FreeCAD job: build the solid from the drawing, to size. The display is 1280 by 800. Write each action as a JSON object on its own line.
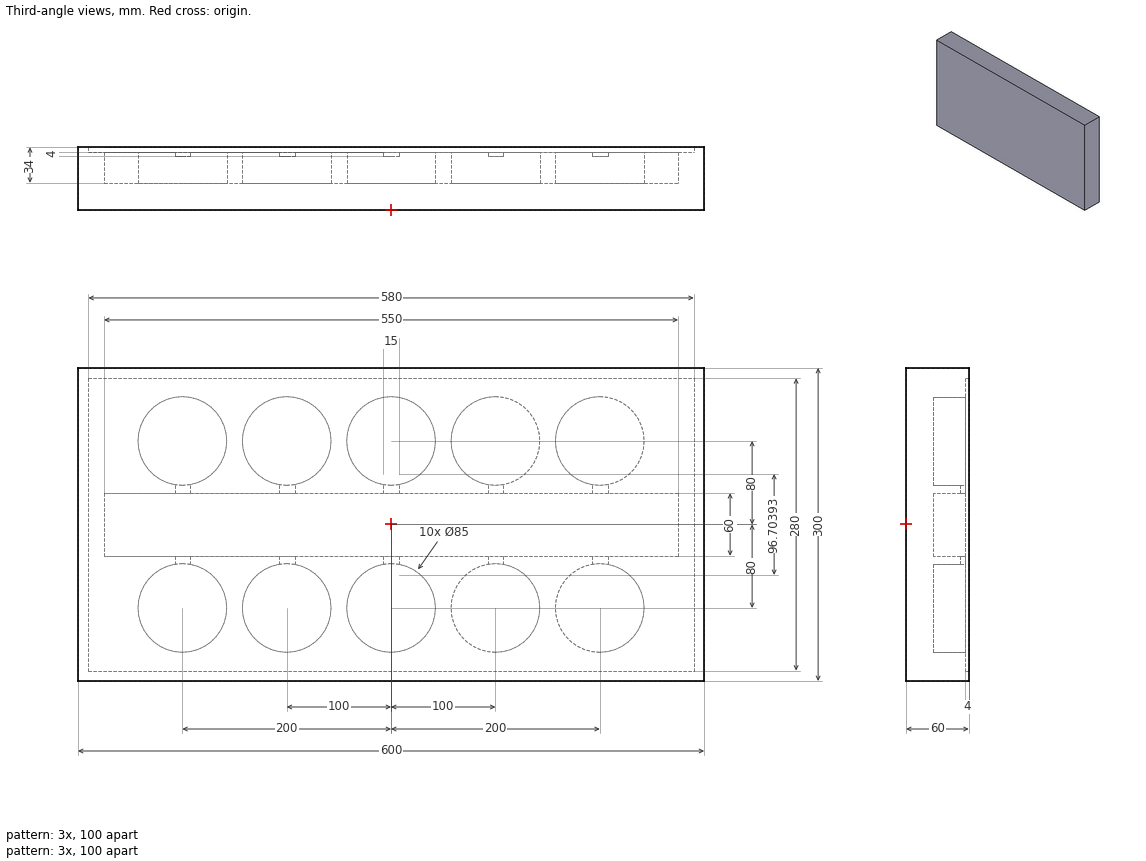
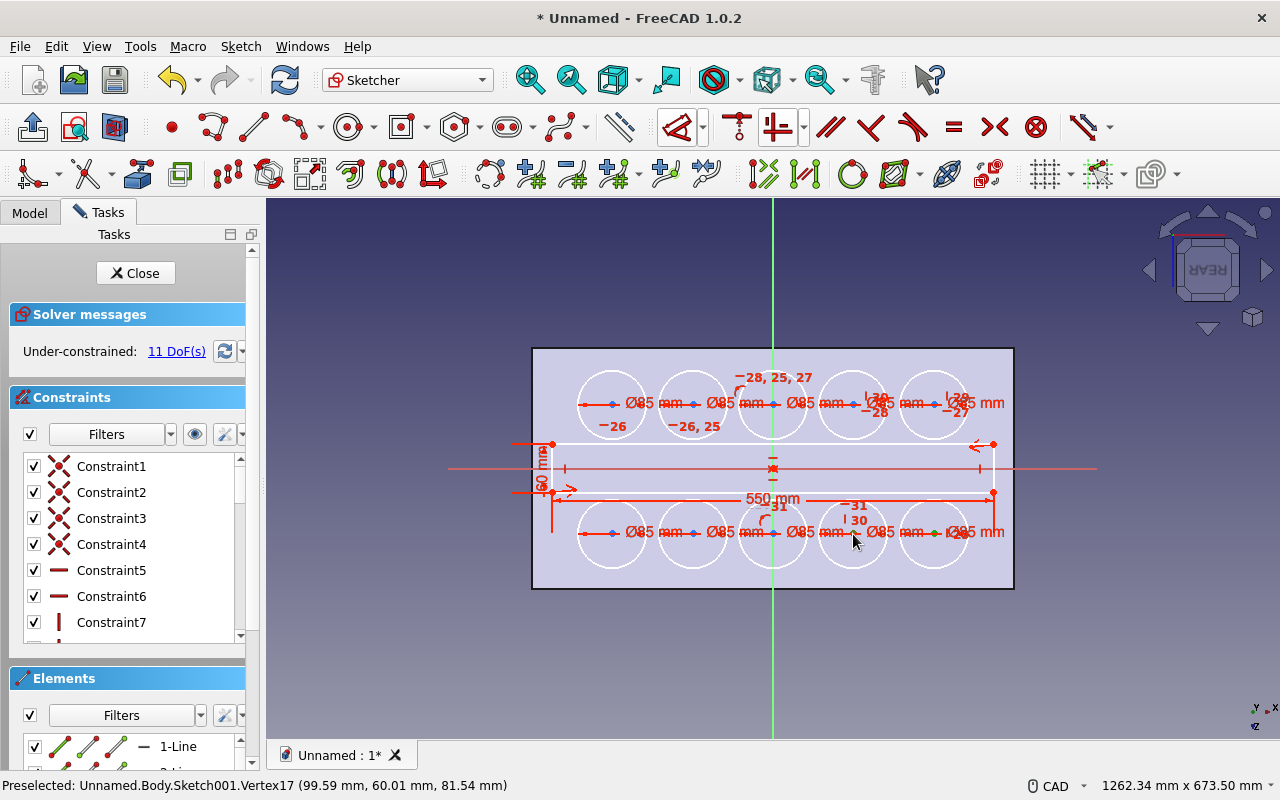
{"action": "left_click", "coordinate": [804, 128]}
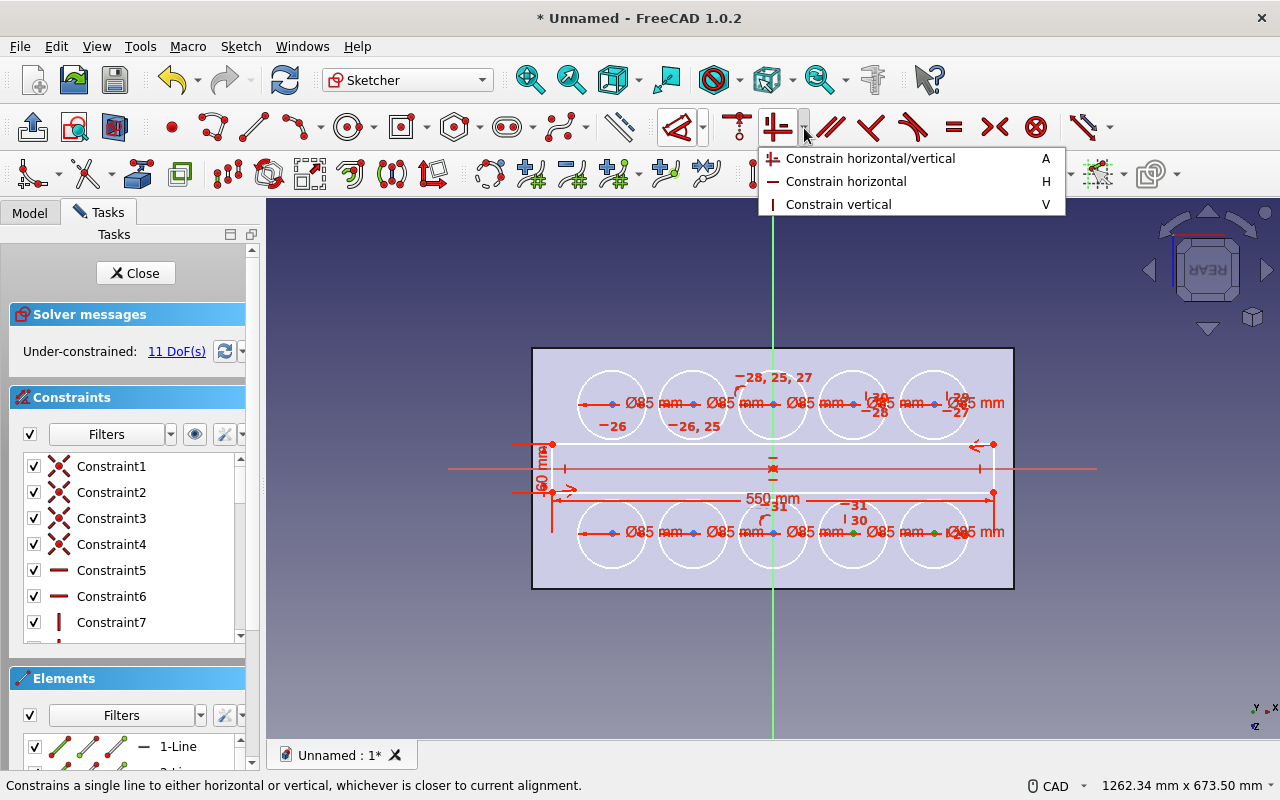
{"action": "left_click", "coordinate": [912, 182]}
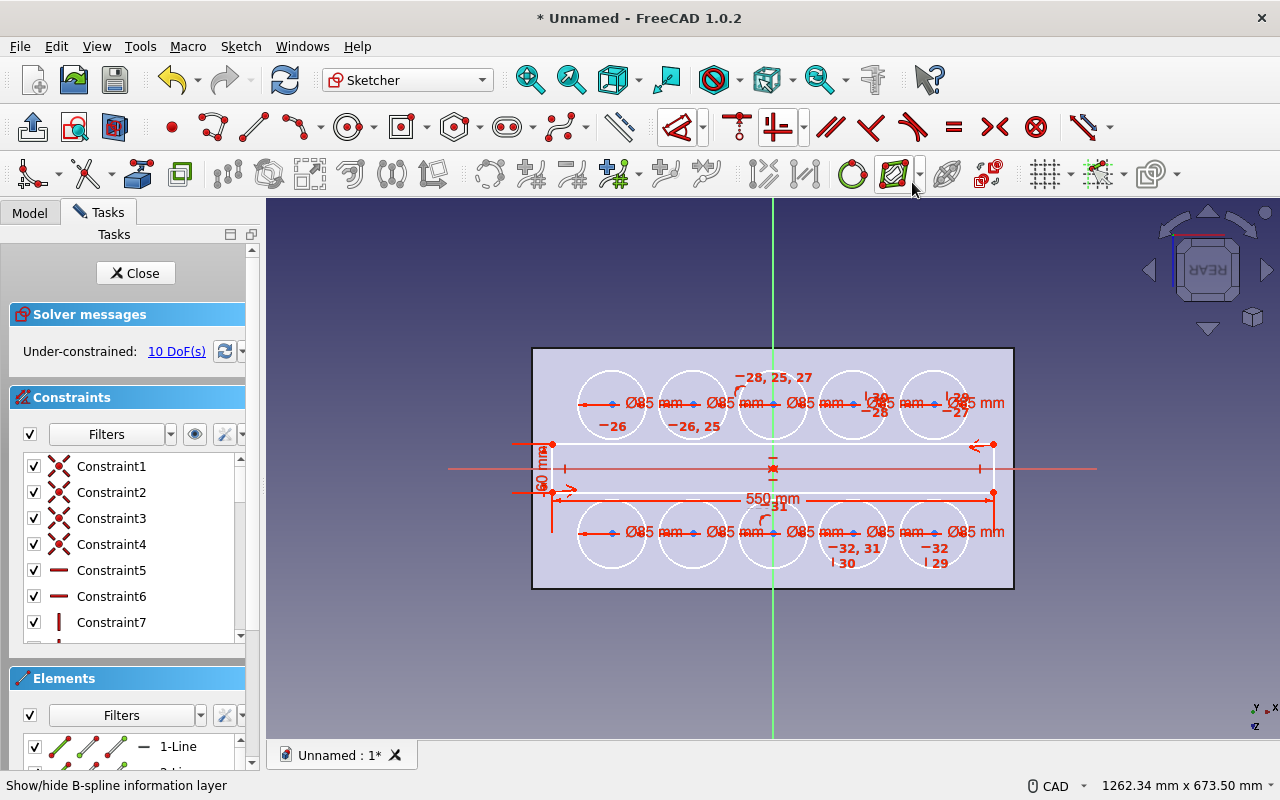
{"action": "left_click", "coordinate": [693, 405]}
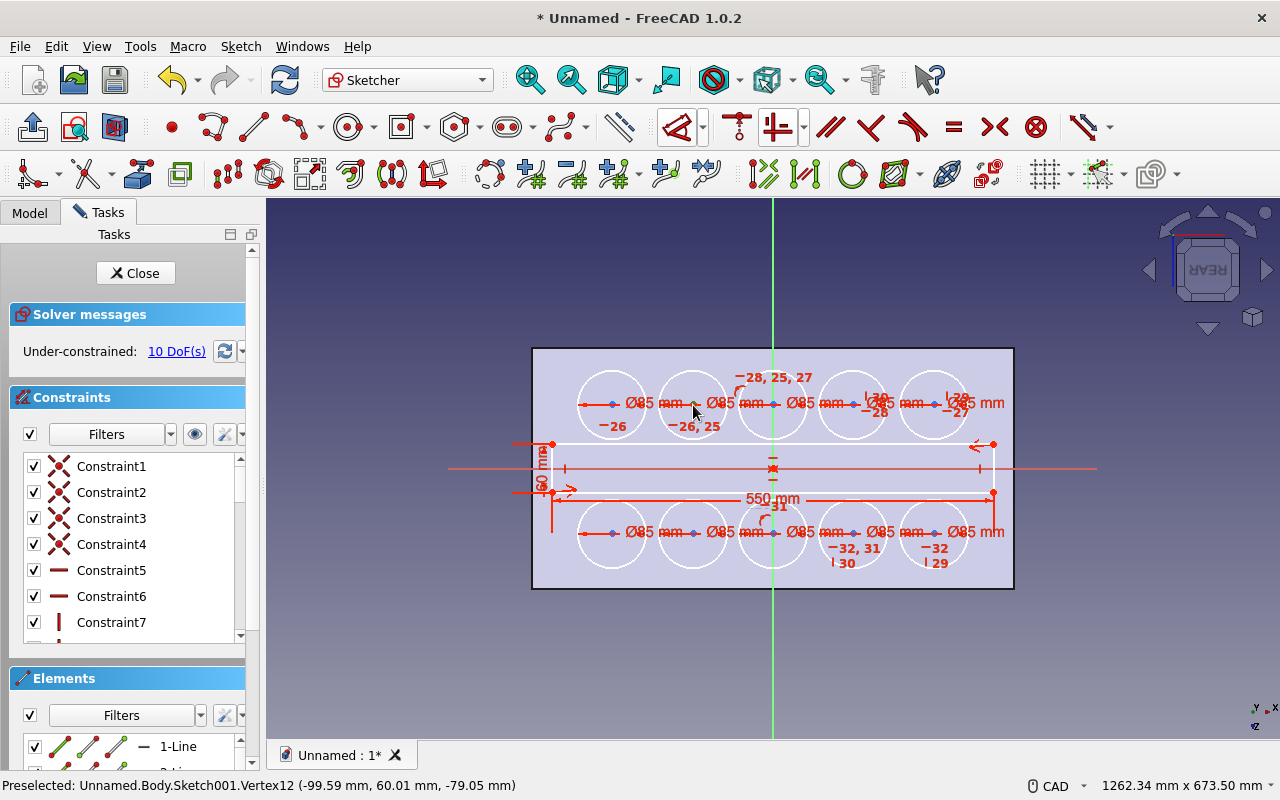
{"action": "left_click", "coordinate": [693, 534]}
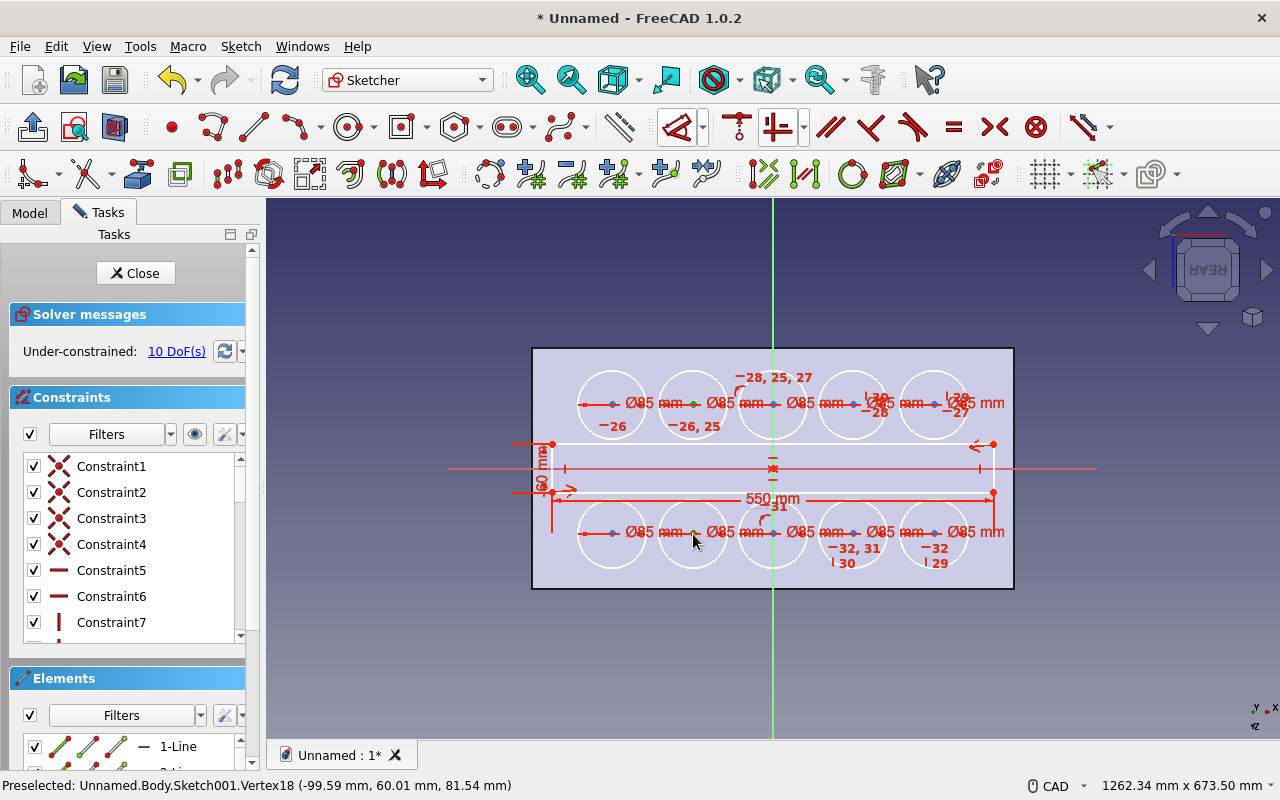
{"action": "key", "text": "v"}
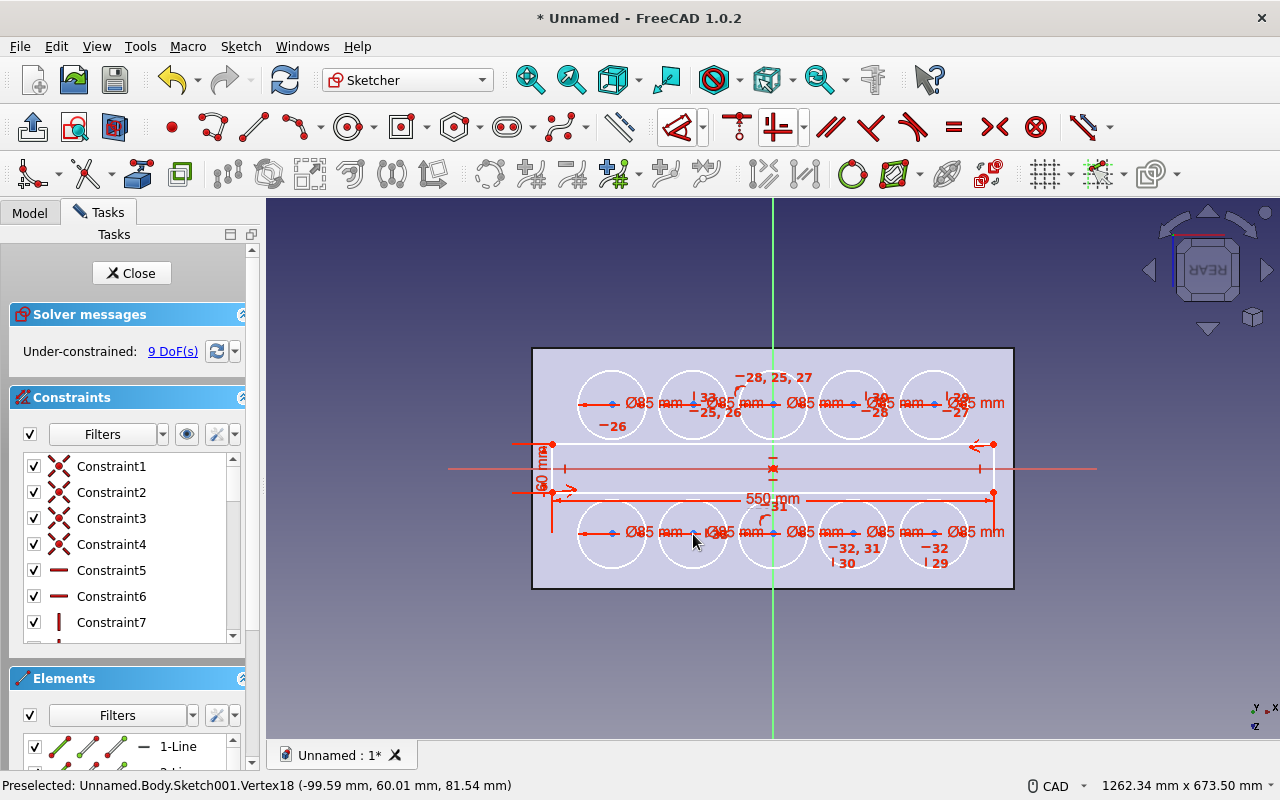
{"action": "left_click", "coordinate": [773, 534]}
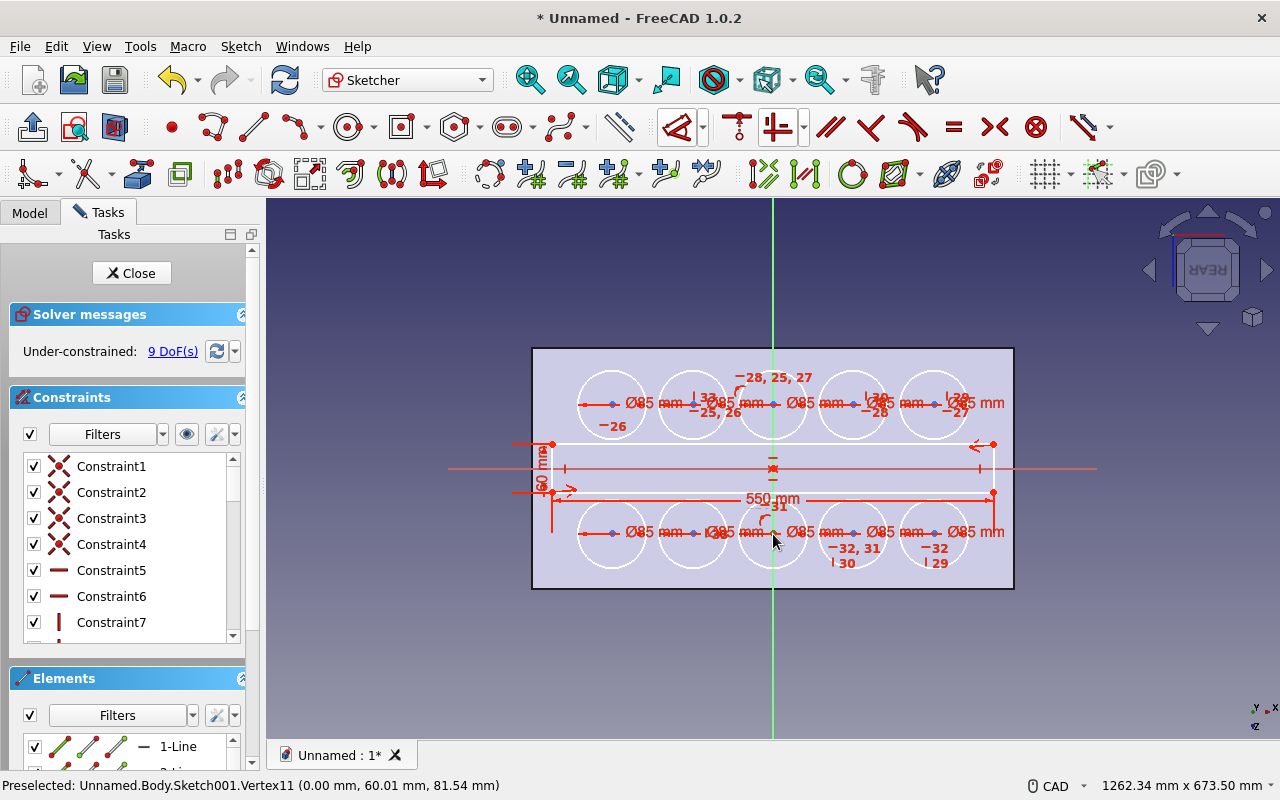
{"action": "left_click", "coordinate": [693, 534]}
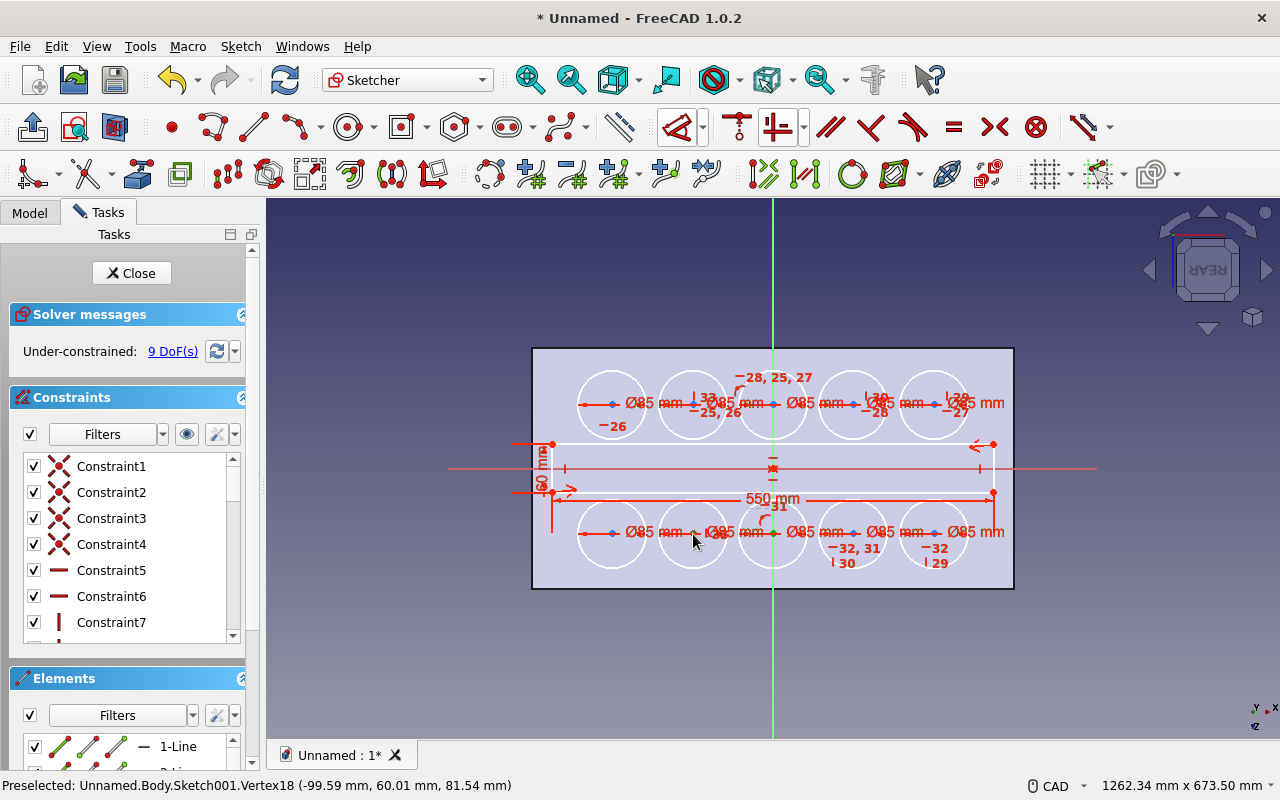
{"action": "left_click", "coordinate": [804, 128]}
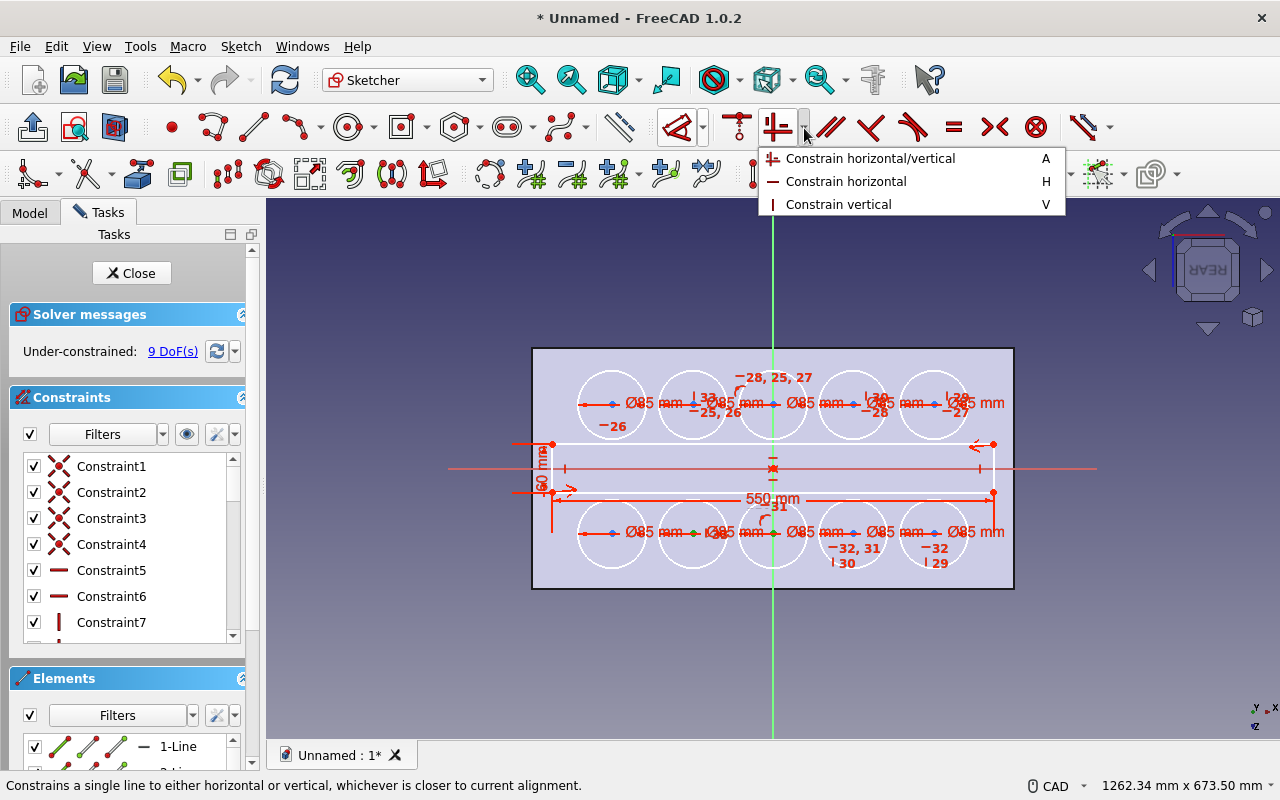
{"action": "left_click", "coordinate": [912, 182]}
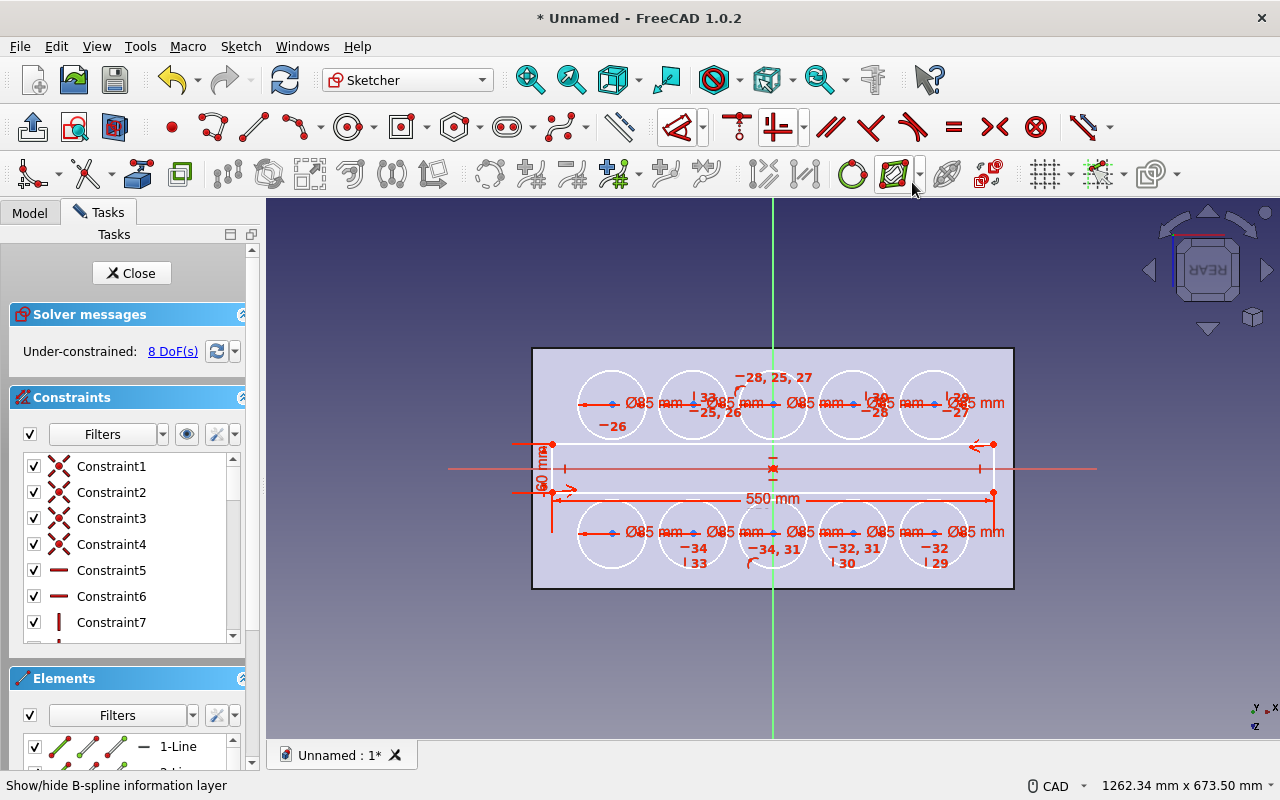
{"action": "left_click", "coordinate": [612, 405]}